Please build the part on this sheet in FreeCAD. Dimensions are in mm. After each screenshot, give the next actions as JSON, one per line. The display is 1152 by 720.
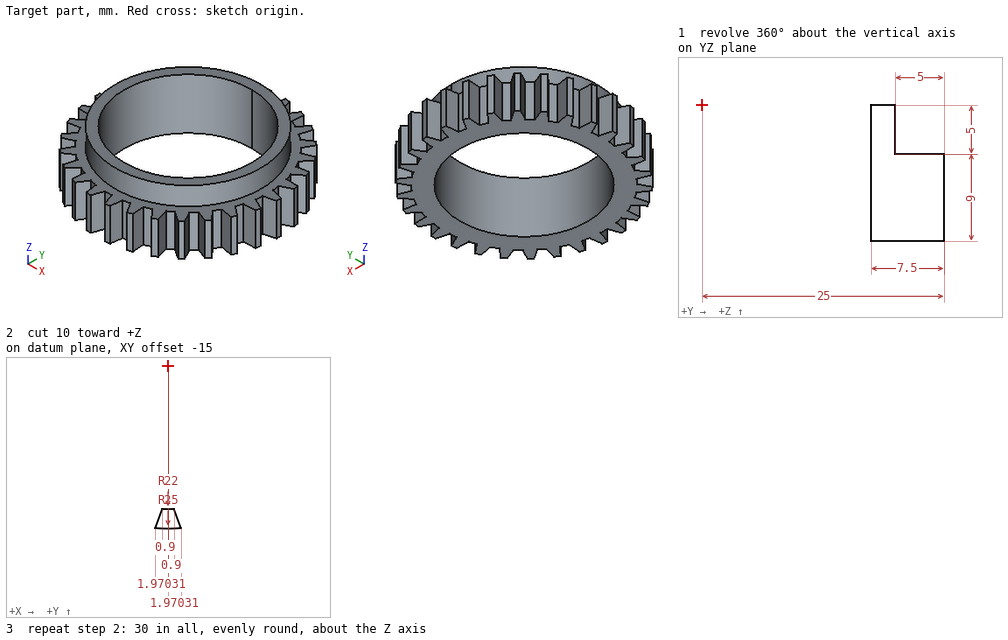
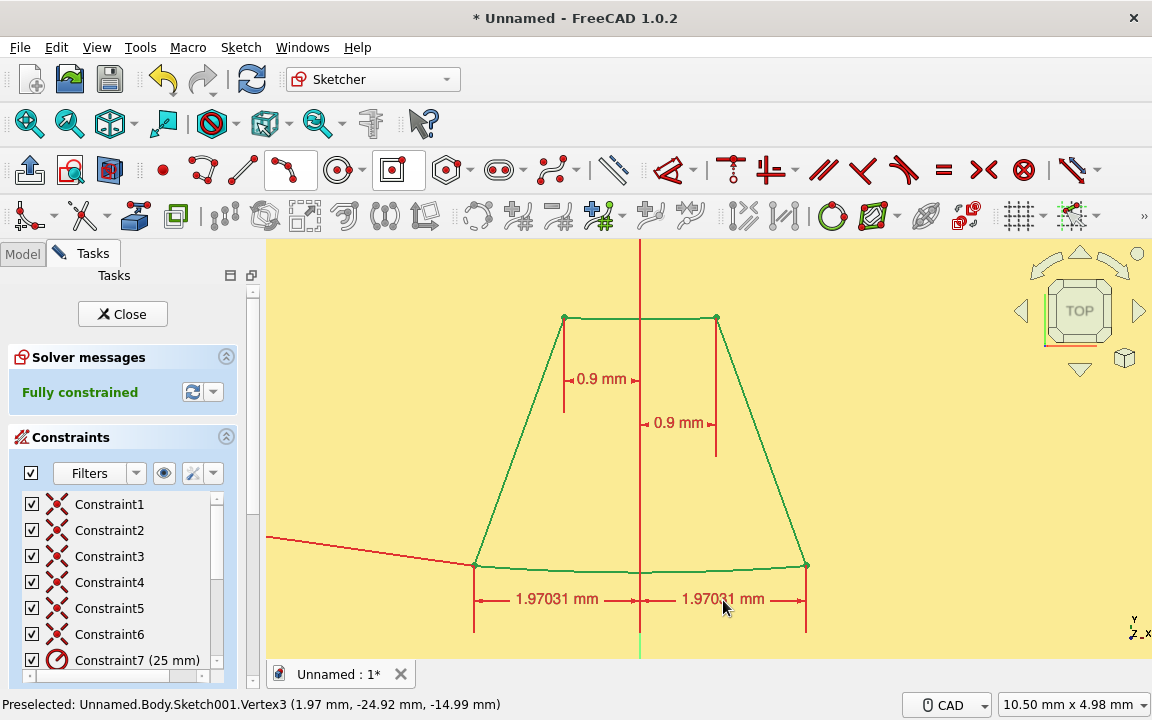
{"action": "left_click", "coordinate": [123, 314]}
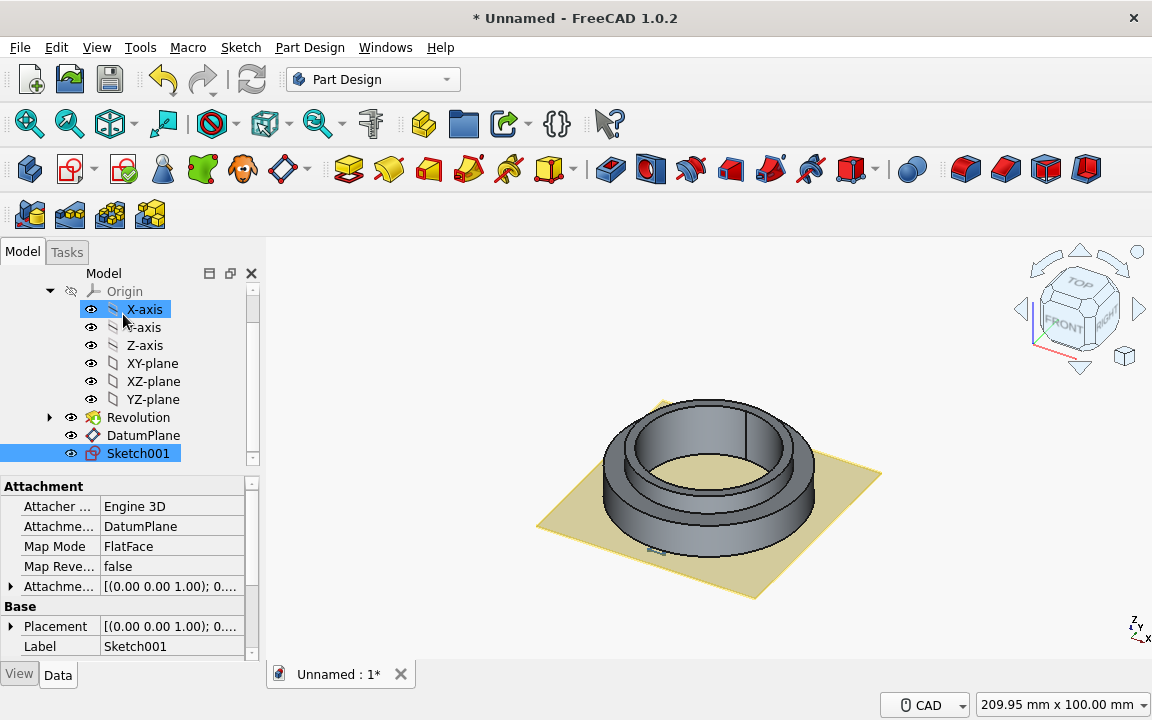
{"action": "left_click", "coordinate": [612, 170]}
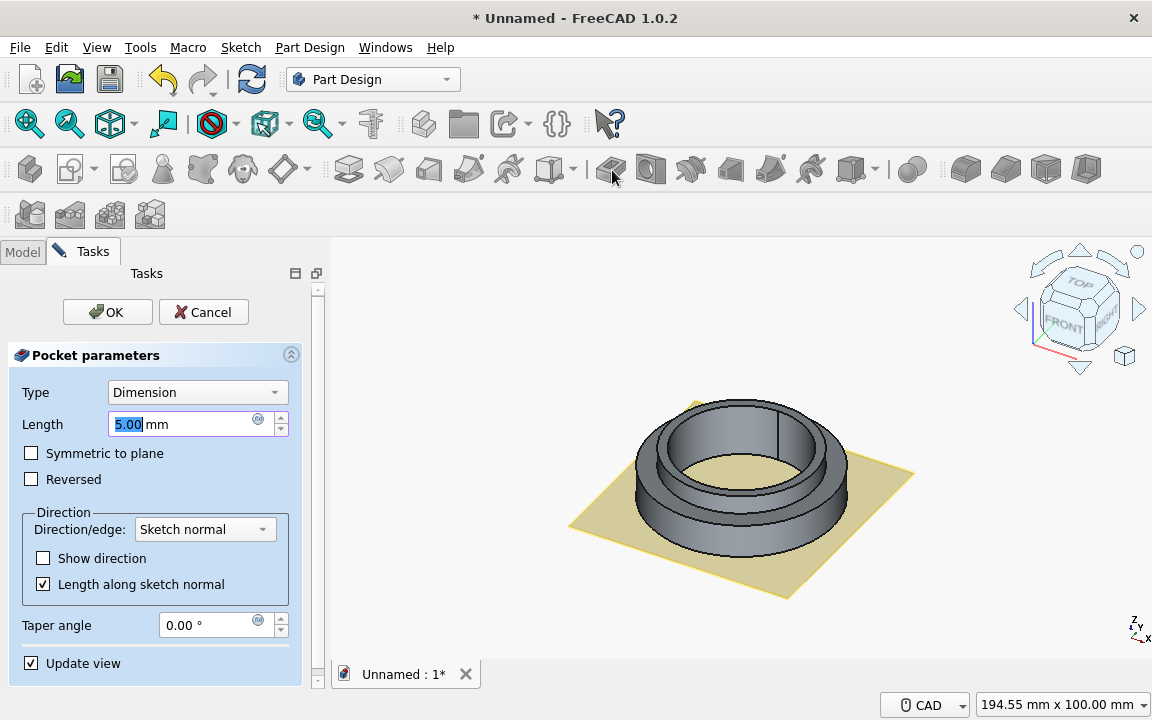
{"action": "type", "text": "10"}
{"action": "key", "text": "Tab"}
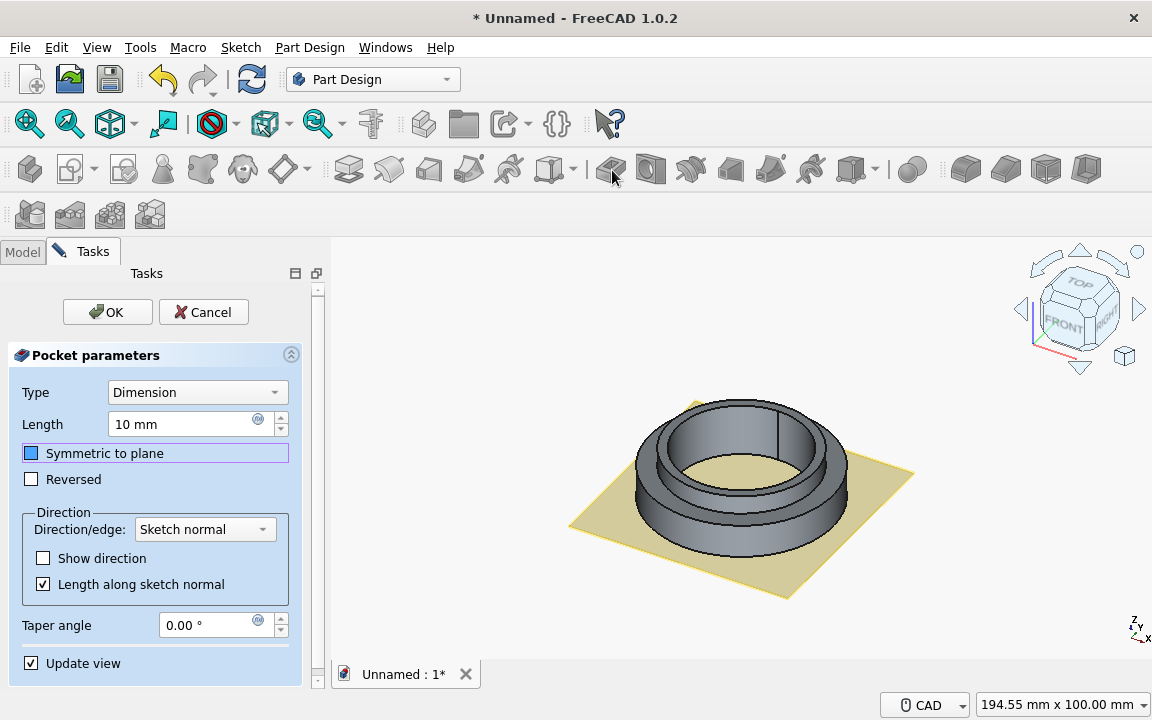
{"action": "left_click", "coordinate": [30, 479]}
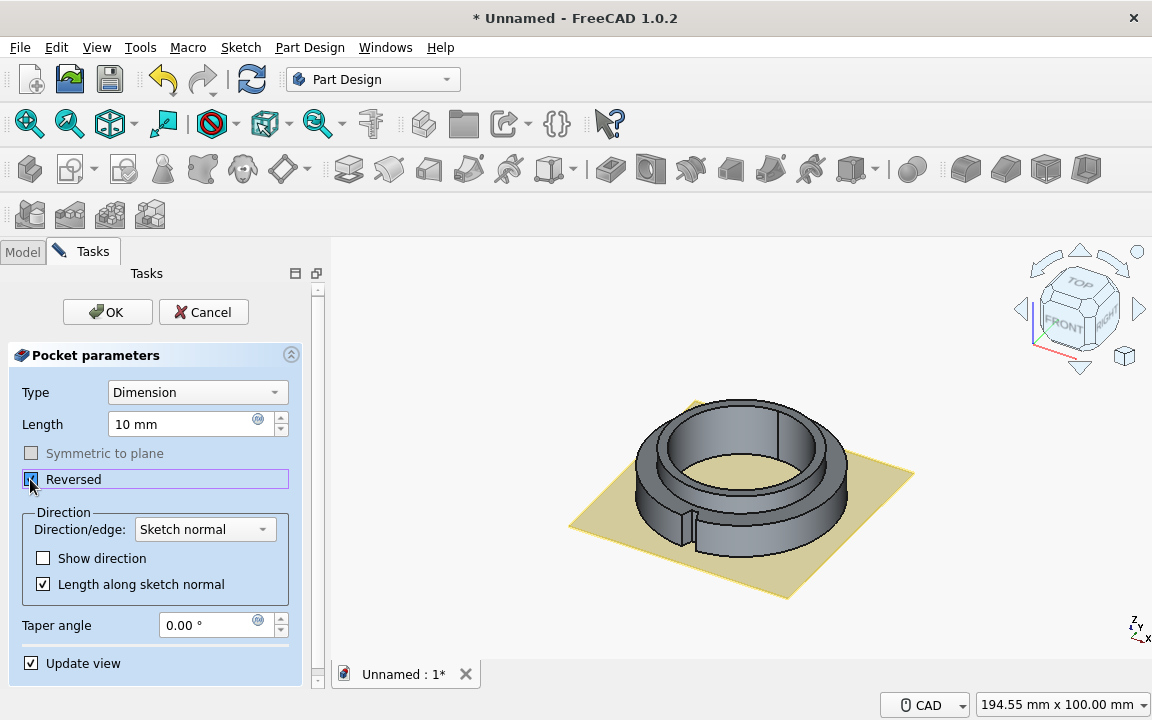
{"action": "left_click", "coordinate": [108, 312]}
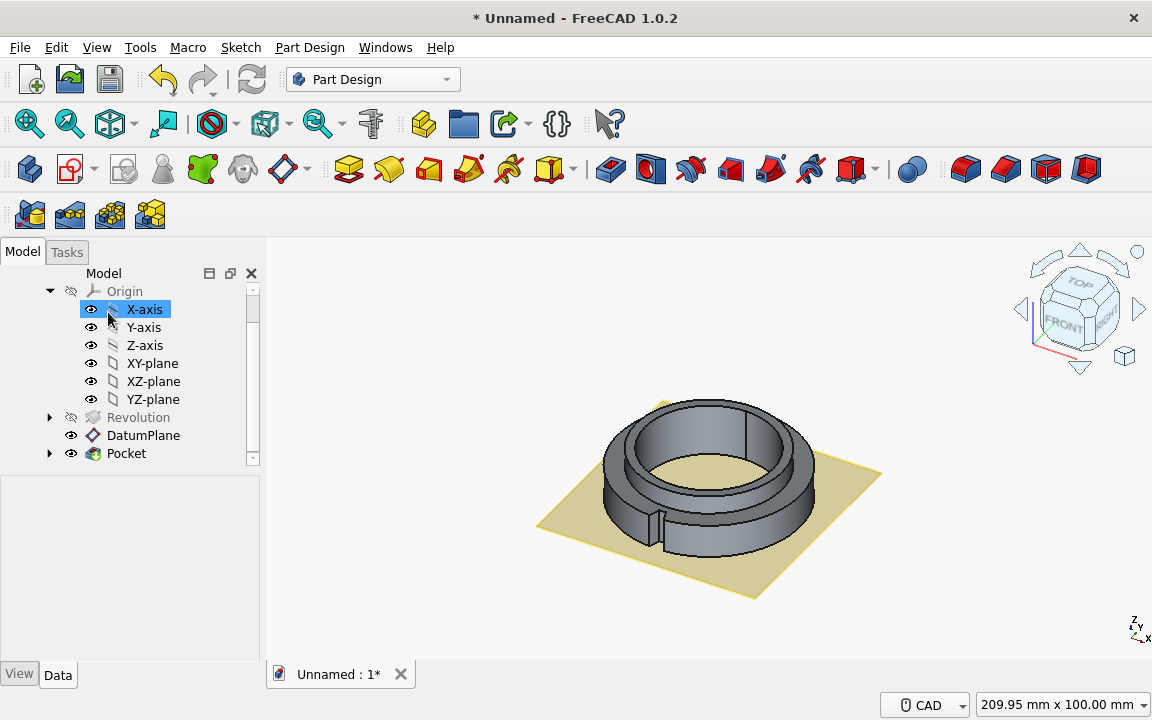
{"action": "left_click", "coordinate": [116, 435]}
{"action": "key", "text": "space"}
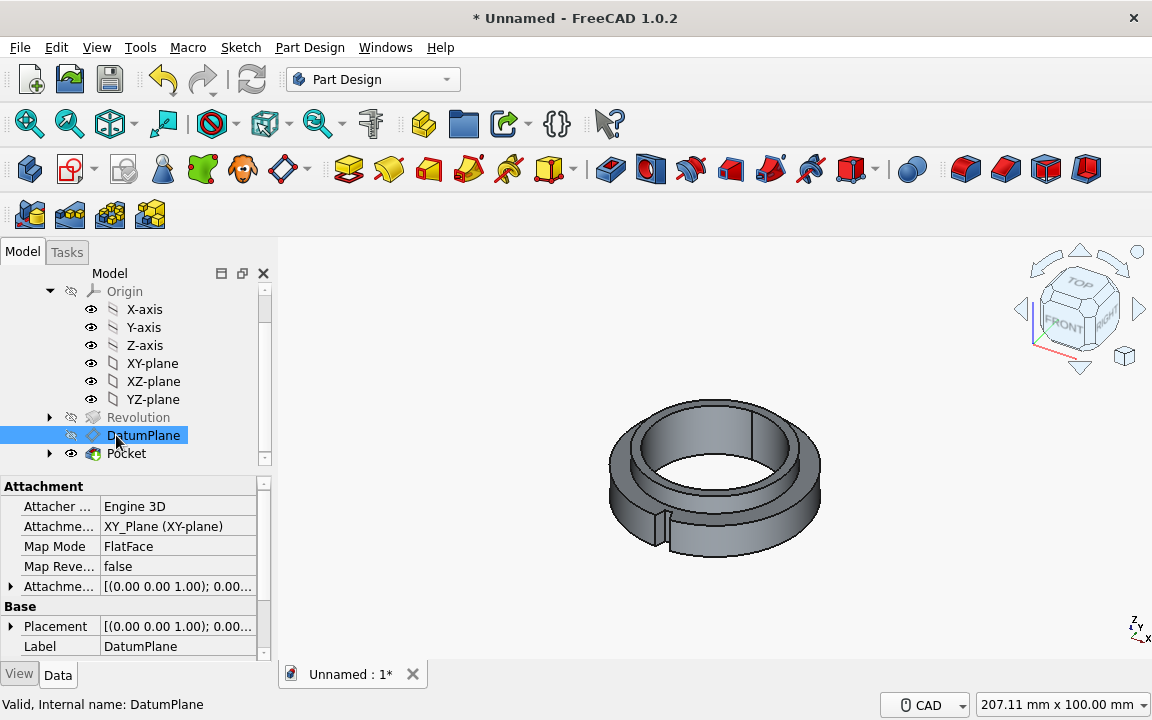
{"action": "left_click", "coordinate": [116, 453]}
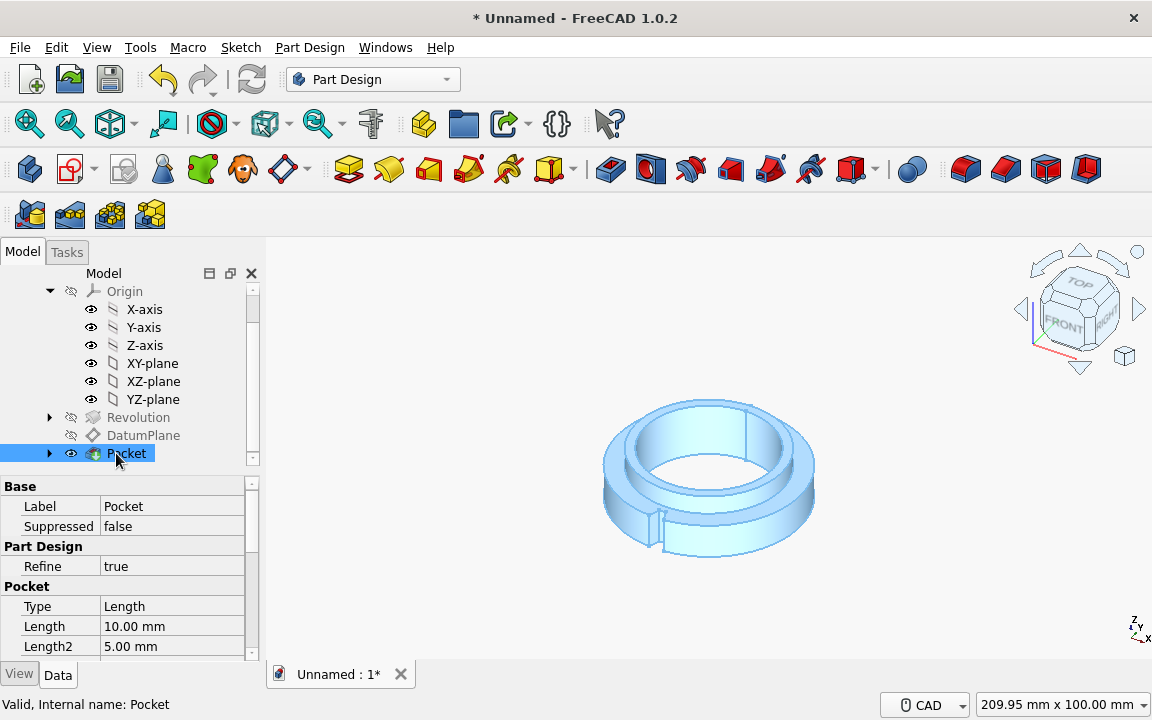
{"action": "left_click", "coordinate": [110, 214]}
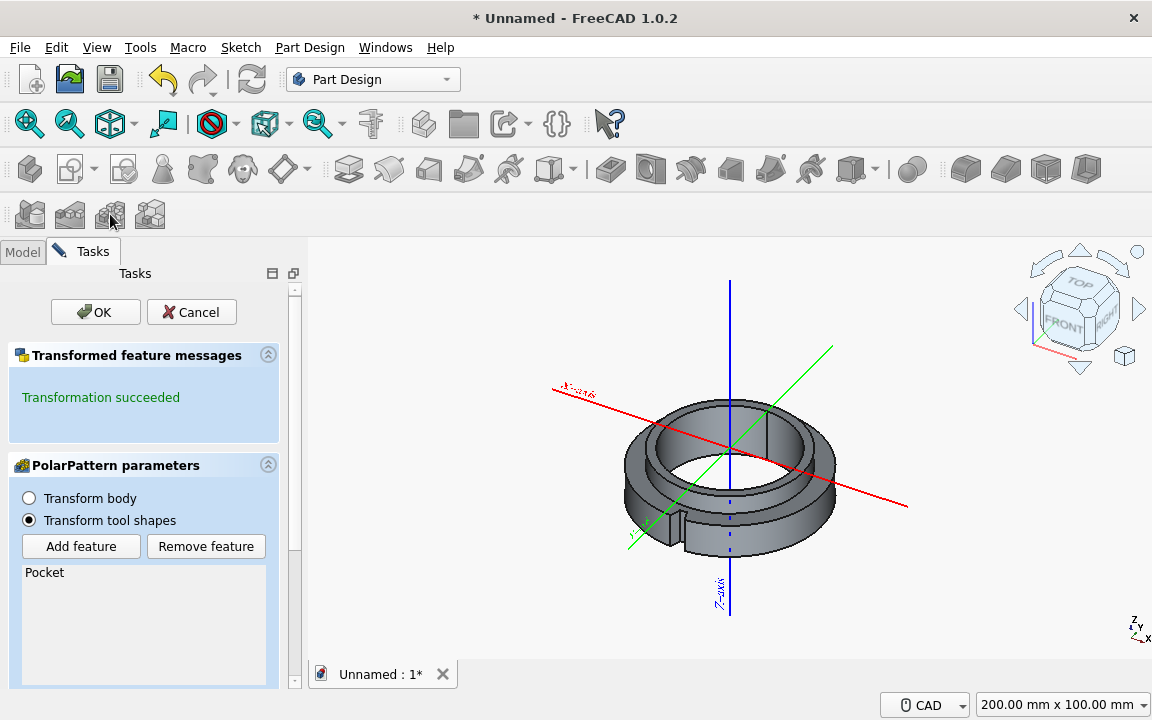
{"action": "scroll", "coordinate": [295, 486], "scroll_direction": "down", "scroll_amount": 2}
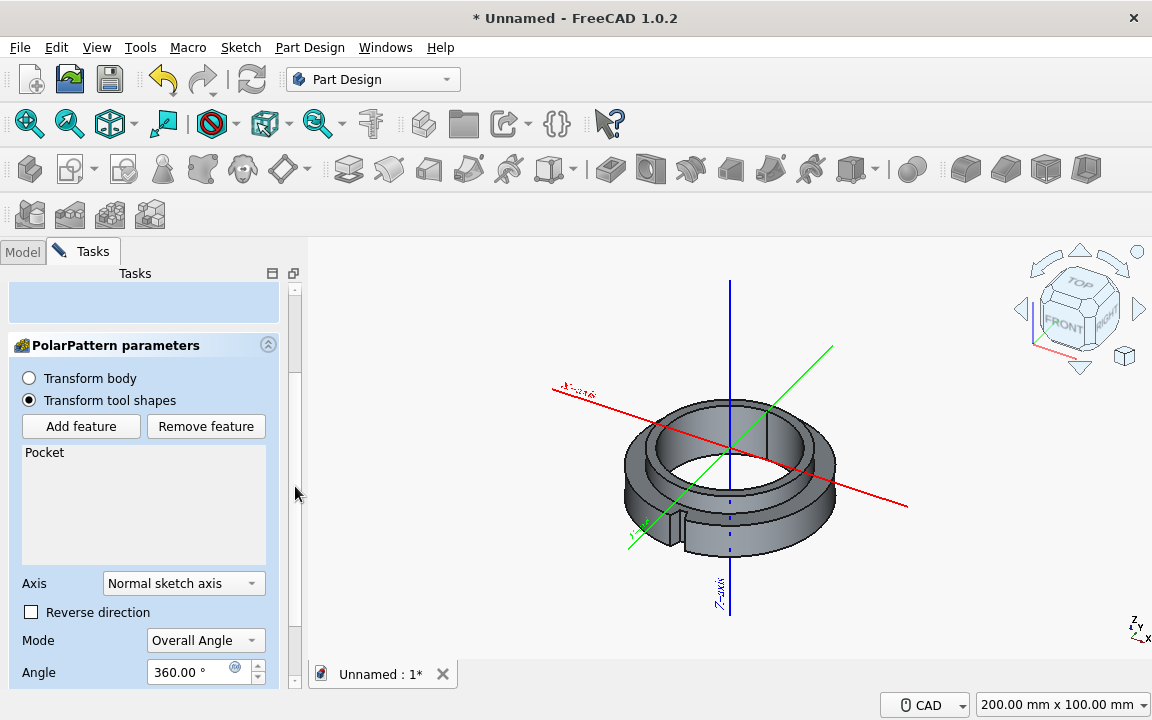
{"action": "left_click", "coordinate": [184, 584]}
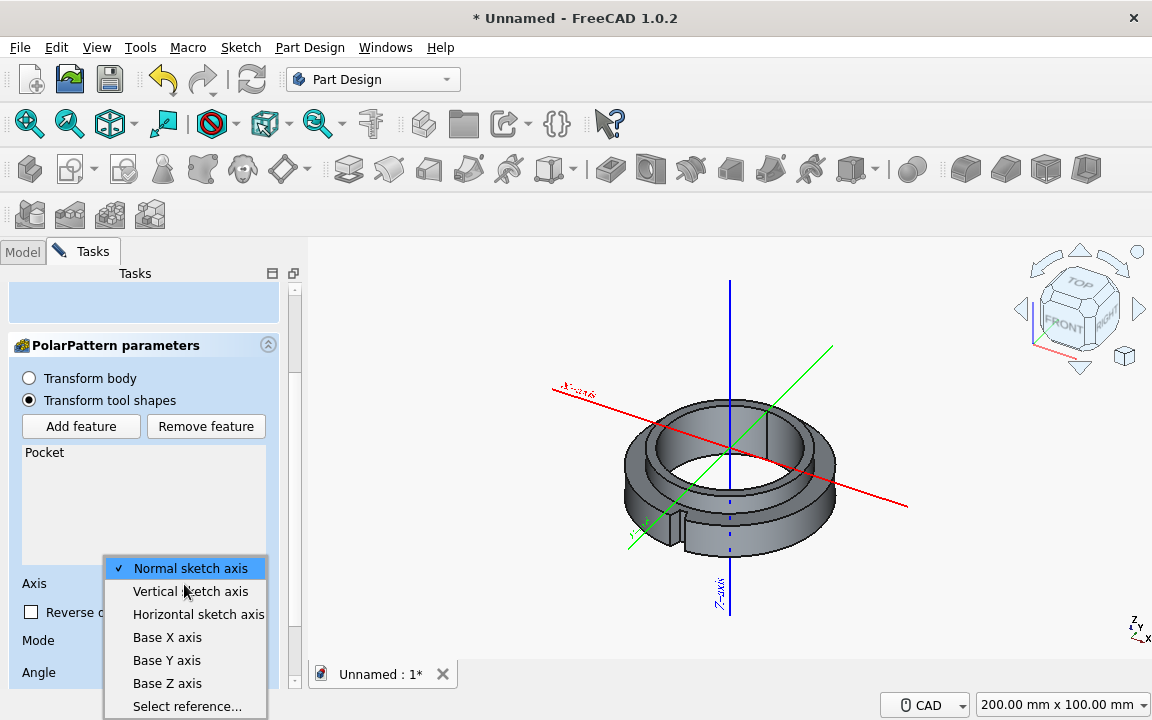
{"action": "left_click", "coordinate": [184, 684]}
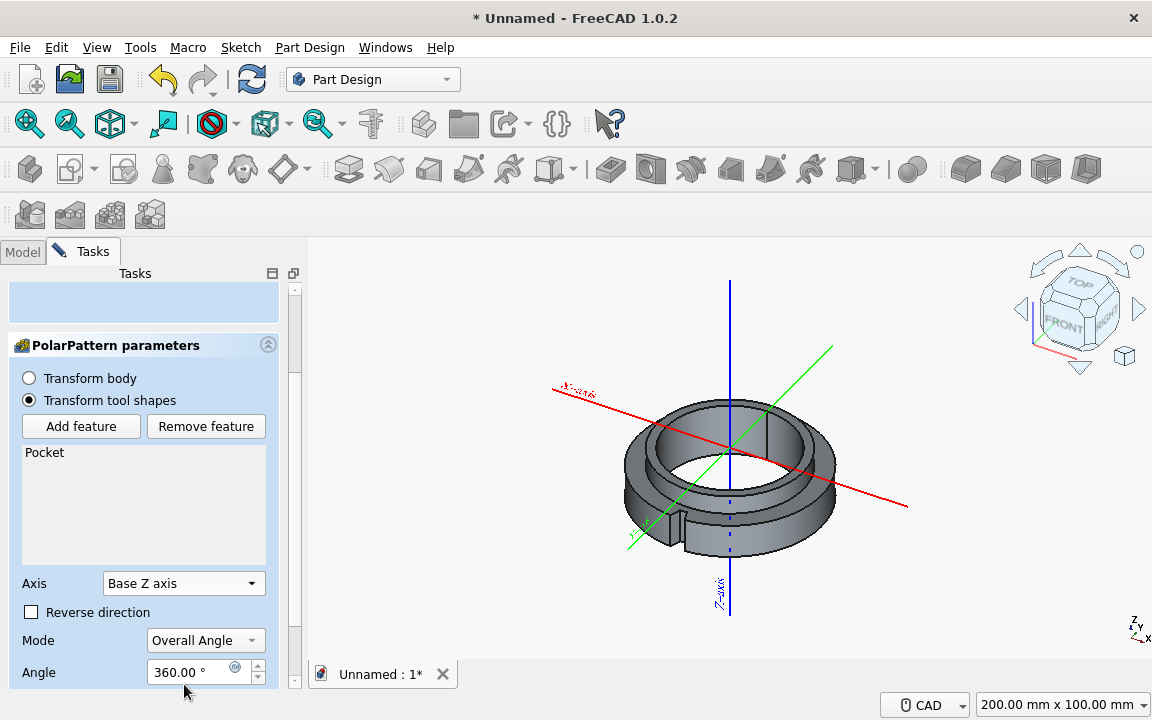
{"action": "scroll", "coordinate": [295, 486], "scroll_direction": "down", "scroll_amount": 2}